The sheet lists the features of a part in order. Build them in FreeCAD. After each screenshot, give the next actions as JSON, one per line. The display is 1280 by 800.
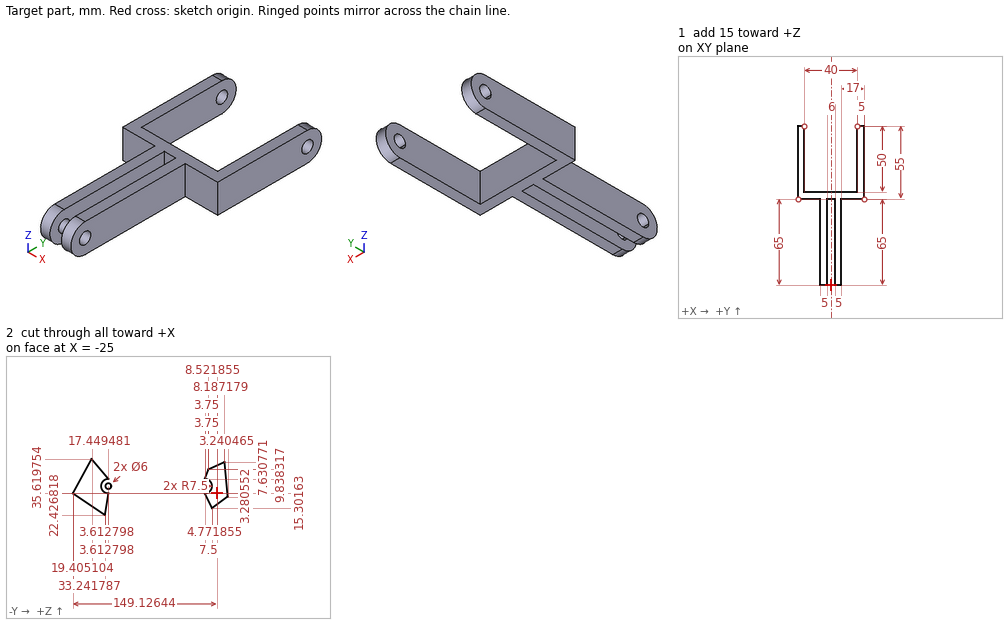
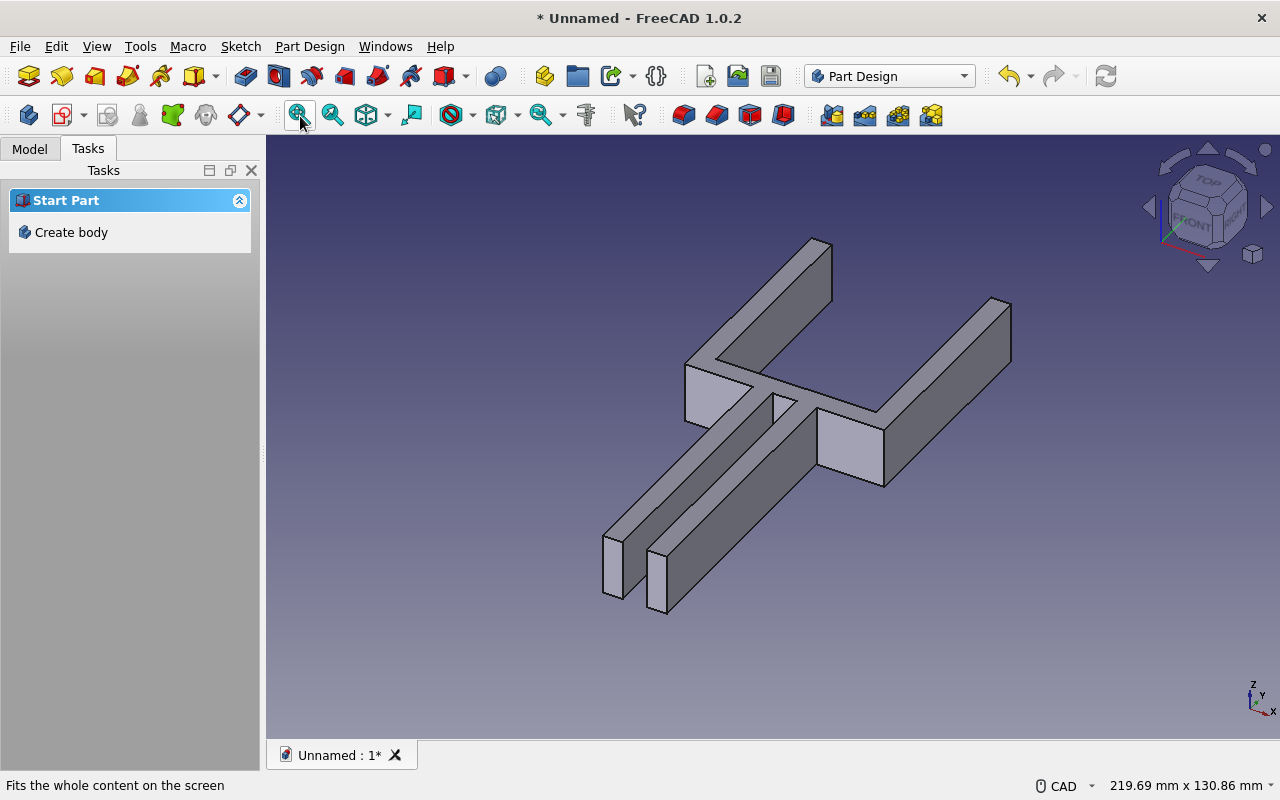
{"action": "key", "text": "6"}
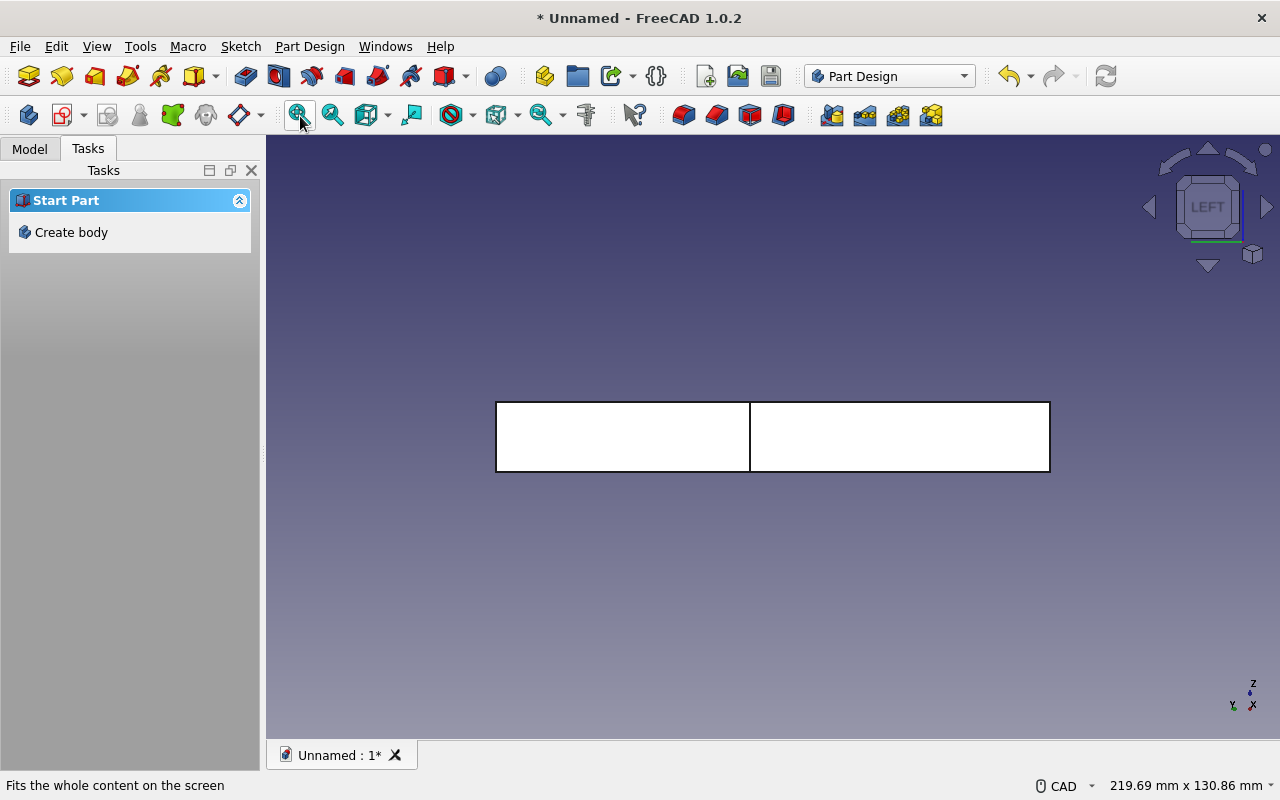
{"action": "left_click", "coordinate": [550, 436]}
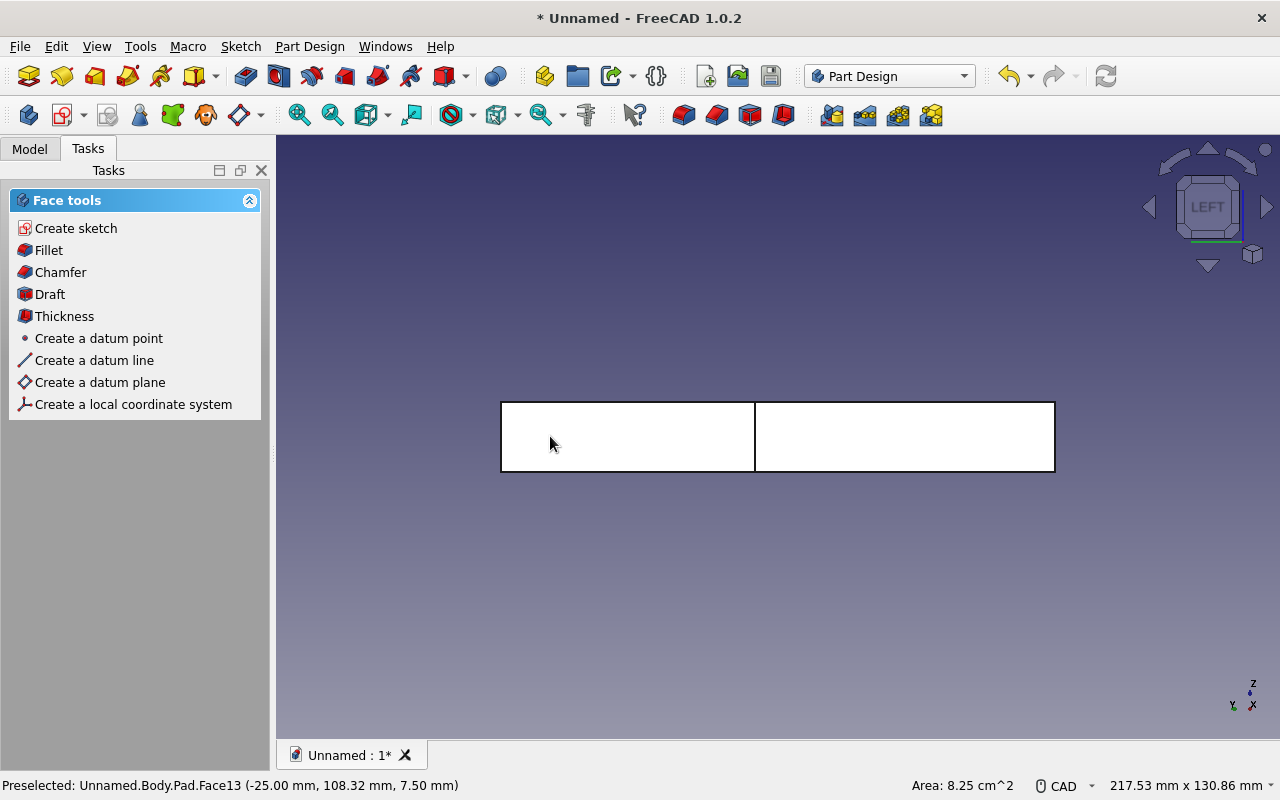
{"action": "left_click", "coordinate": [62, 116]}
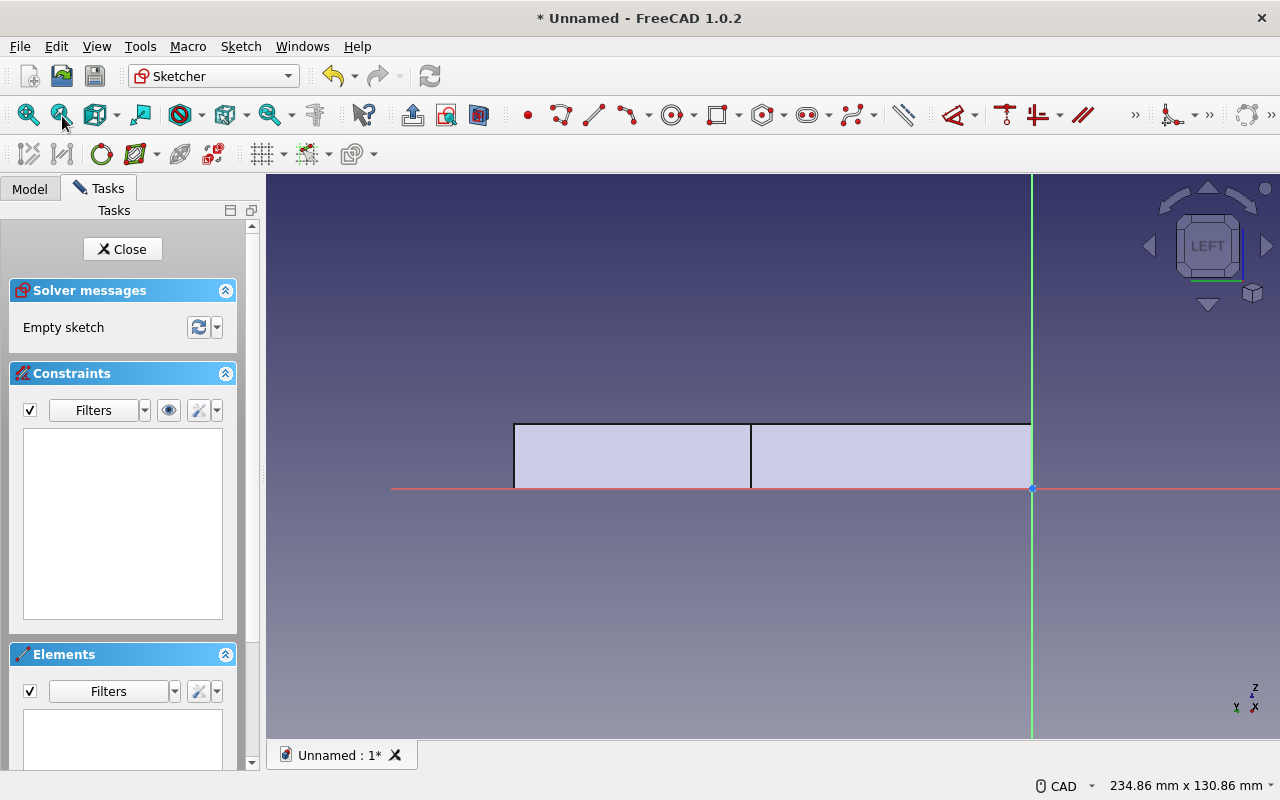
{"action": "key", "text": "g m"}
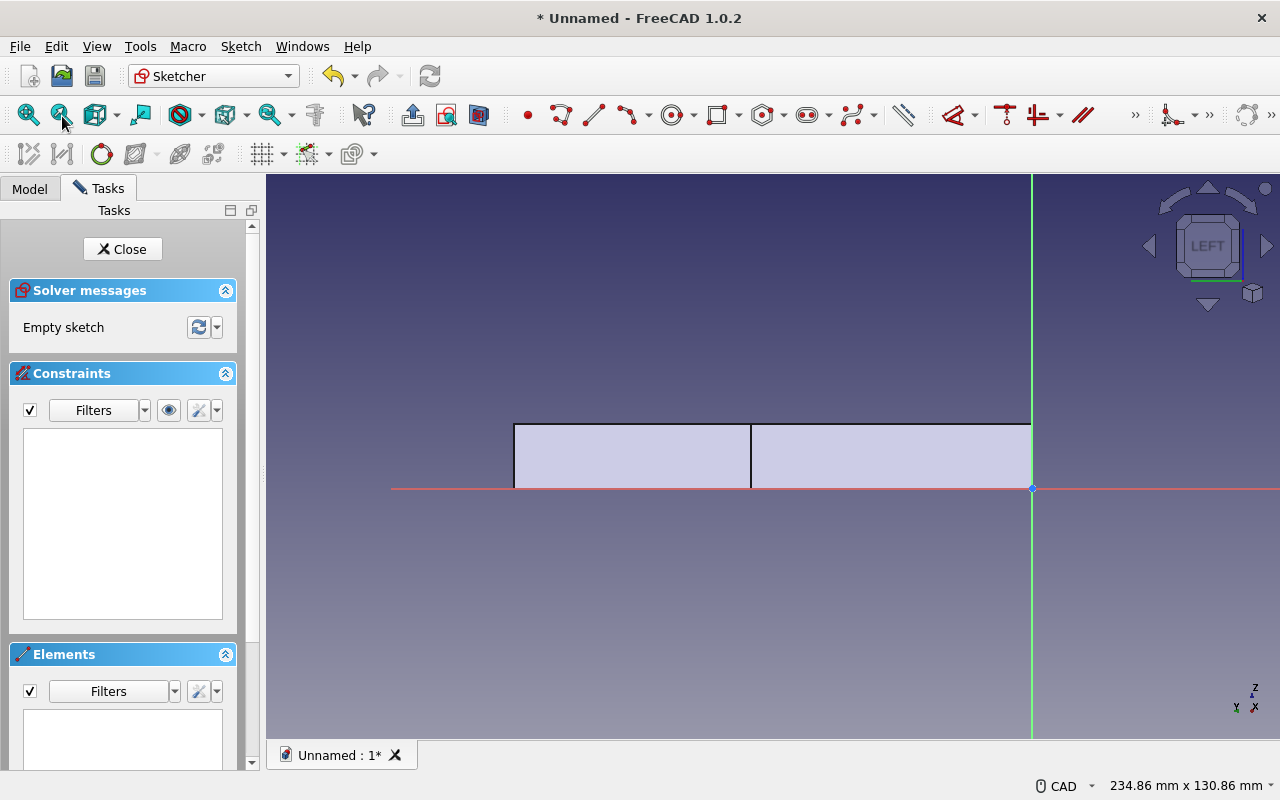
{"action": "left_click", "coordinate": [547, 424]}
{"action": "left_click", "coordinate": [472, 335]}
{"action": "left_click", "coordinate": [388, 489]}
{"action": "left_click", "coordinate": [532, 586]}
{"action": "left_click", "coordinate": [547, 489]}
{"action": "right_click", "coordinate": [547, 489]}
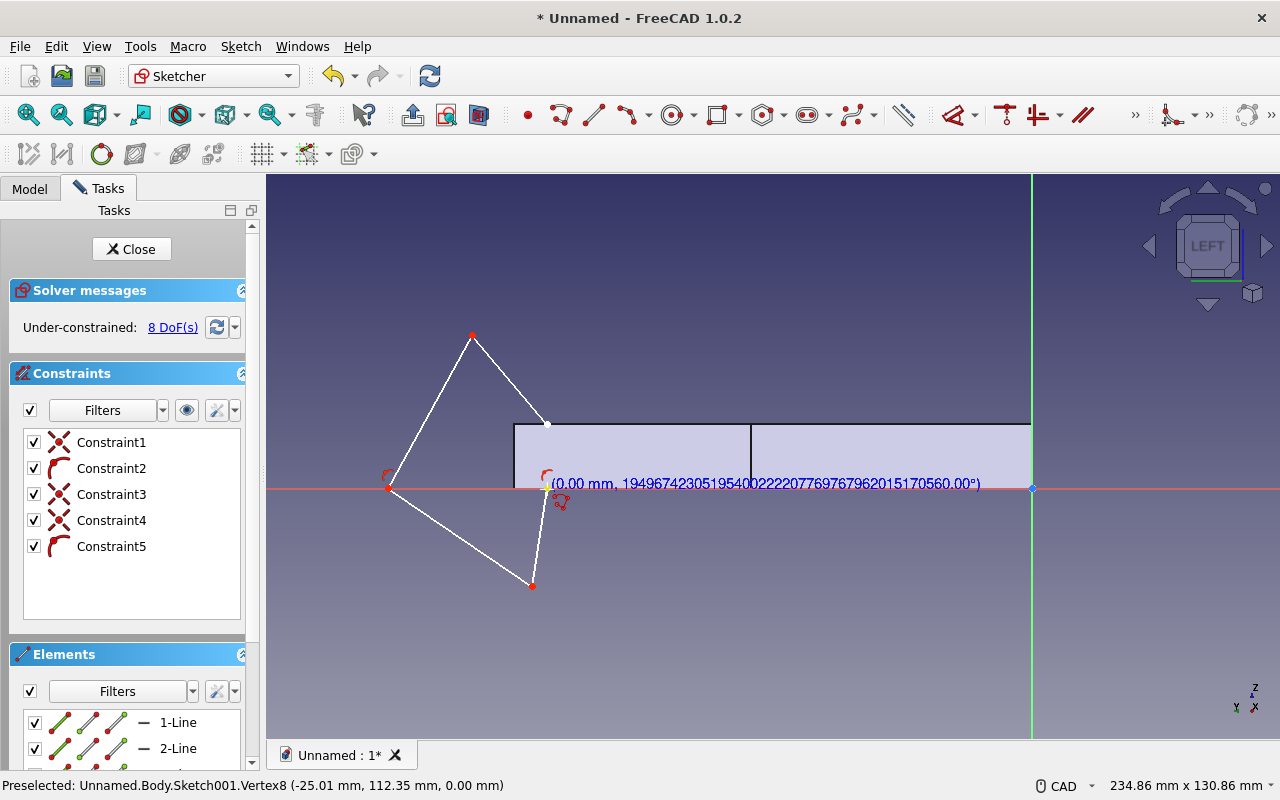
{"action": "key", "text": "g 3 a"}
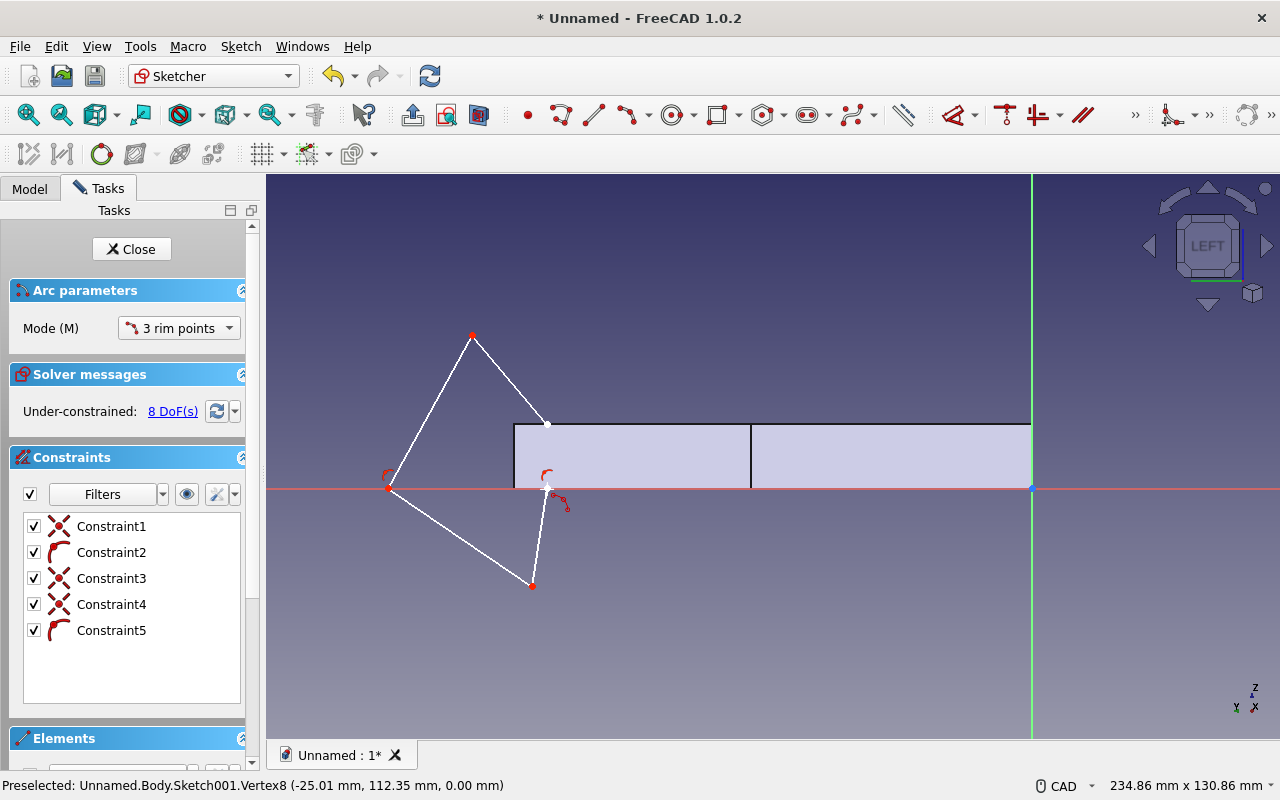
{"action": "left_click", "coordinate": [547, 489]}
{"action": "left_click", "coordinate": [547, 425]}
{"action": "left_click", "coordinate": [515, 456]}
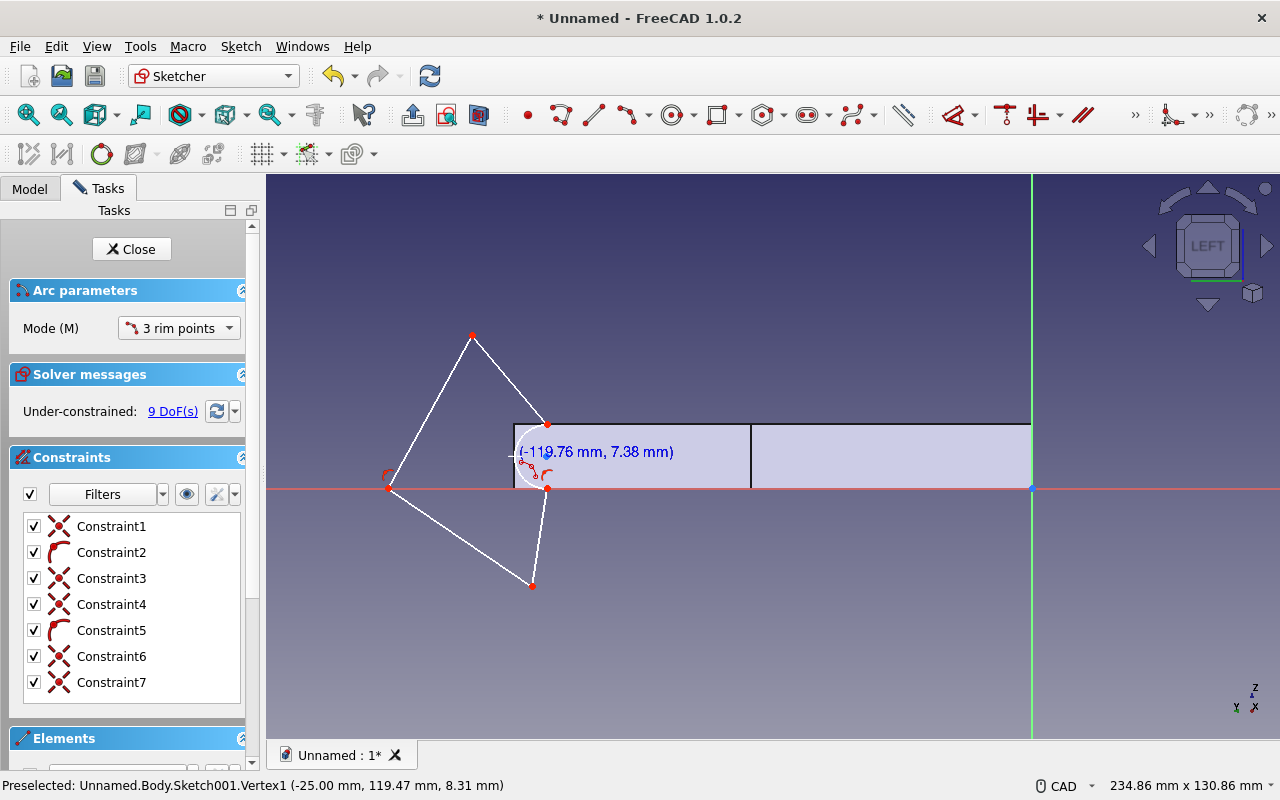
{"action": "left_click", "coordinate": [561, 116]}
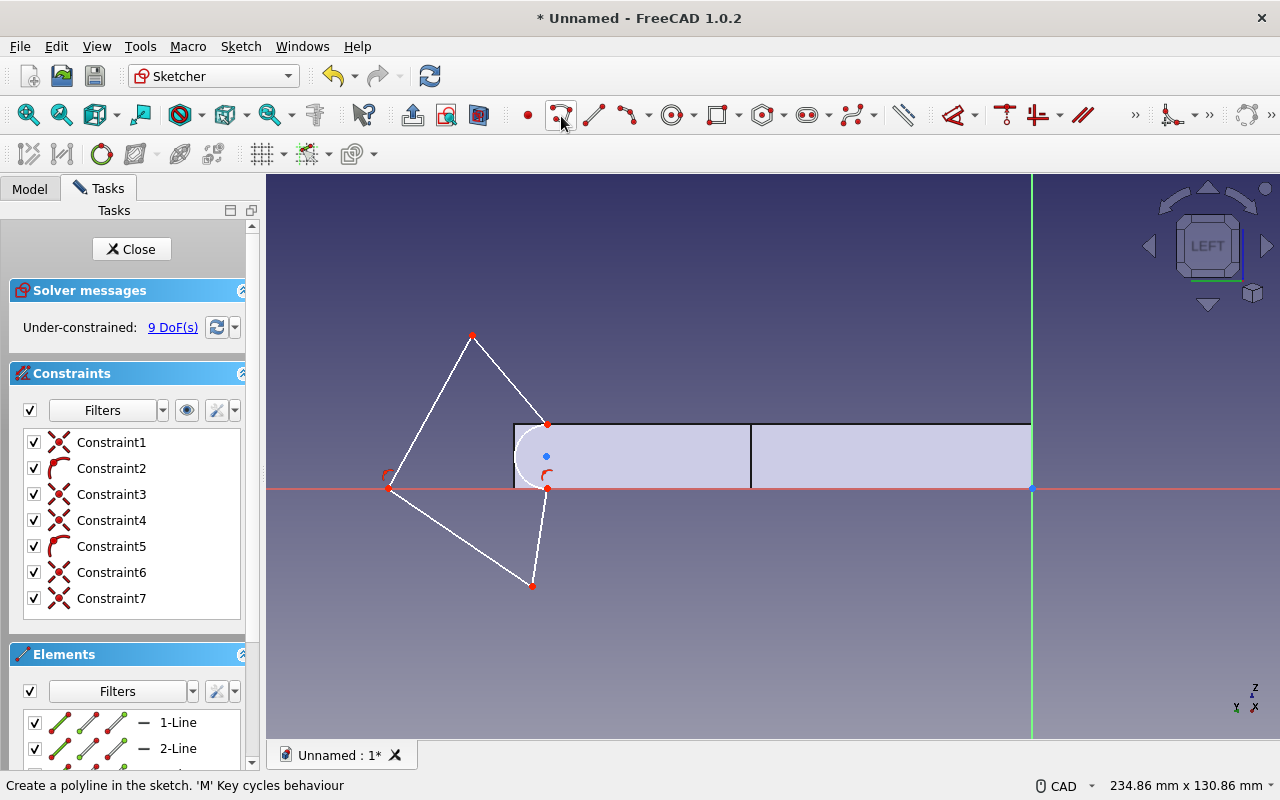
{"action": "left_click", "coordinate": [979, 489]}
{"action": "left_click", "coordinate": [1011, 555]}
{"action": "left_click", "coordinate": [1081, 503]}
{"action": "left_click", "coordinate": [1067, 349]}
{"action": "left_click", "coordinate": [995, 382]}
{"action": "left_click", "coordinate": [979, 424]}
{"action": "right_click", "coordinate": [979, 424]}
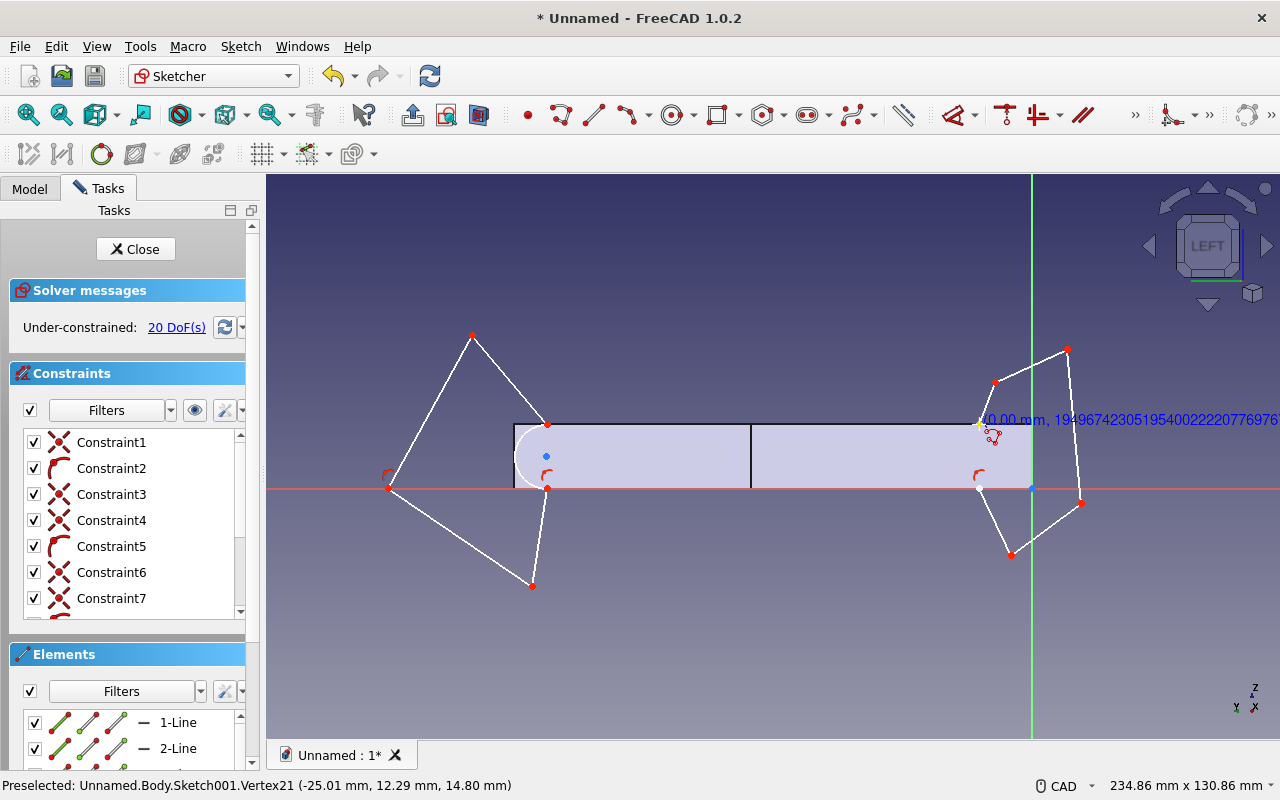
{"action": "left_click", "coordinate": [626, 116]}